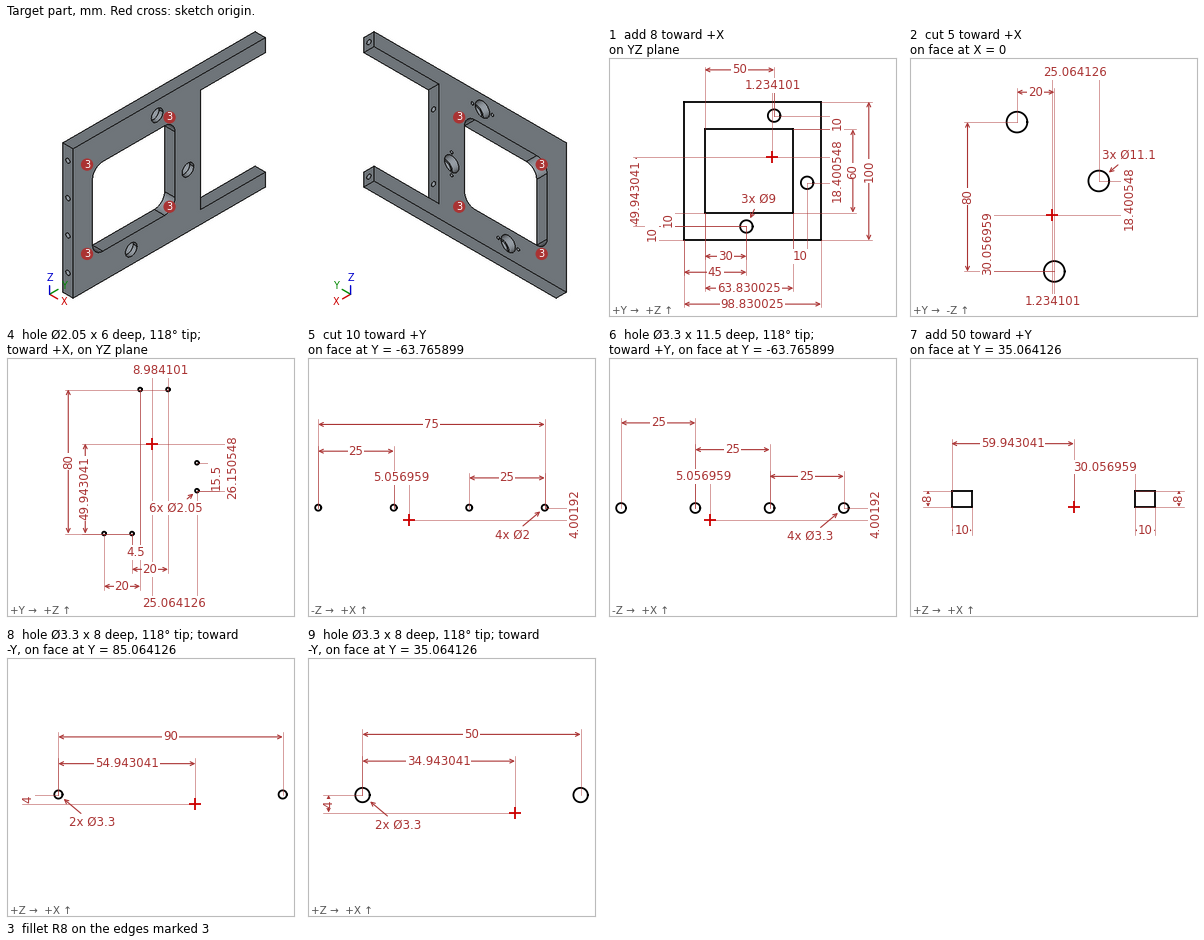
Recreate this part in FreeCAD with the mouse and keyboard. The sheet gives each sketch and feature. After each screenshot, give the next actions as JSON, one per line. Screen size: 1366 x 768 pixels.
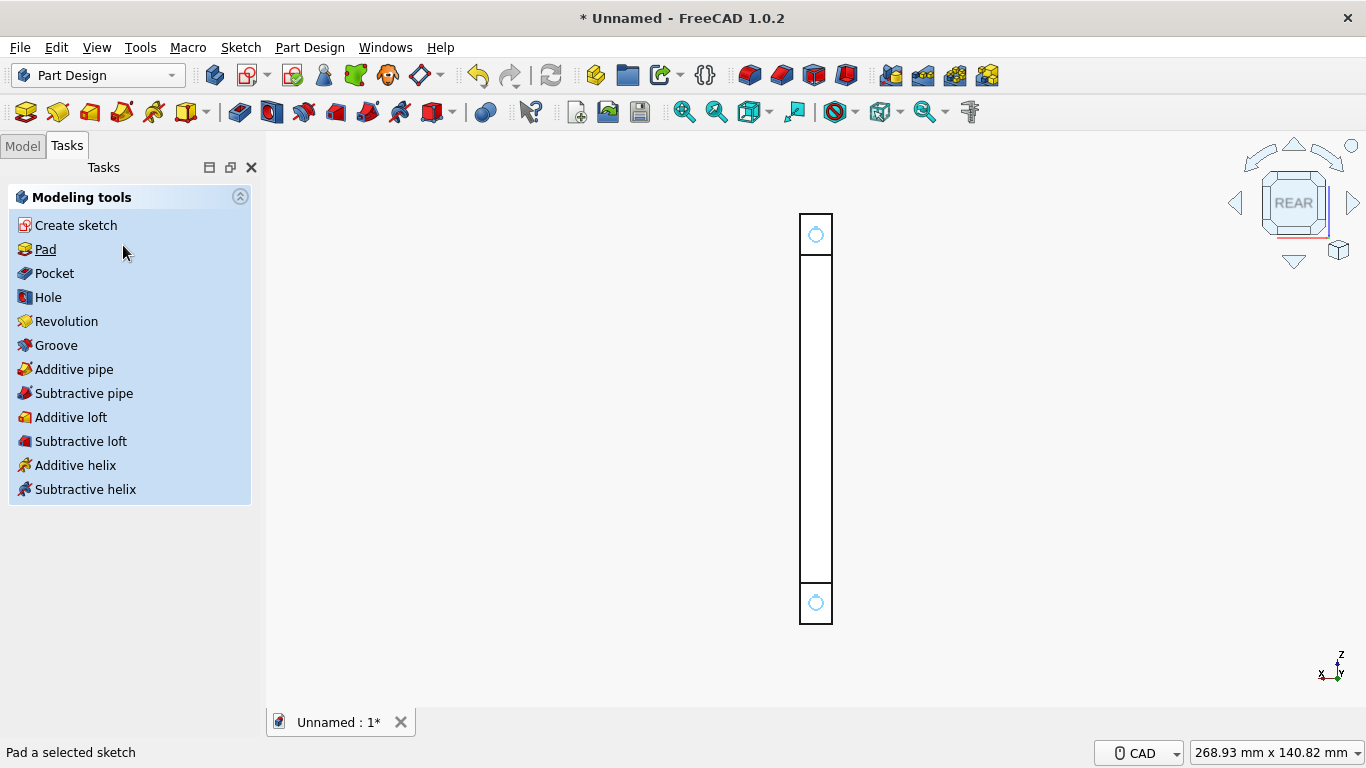
{"action": "left_click", "coordinate": [272, 112]}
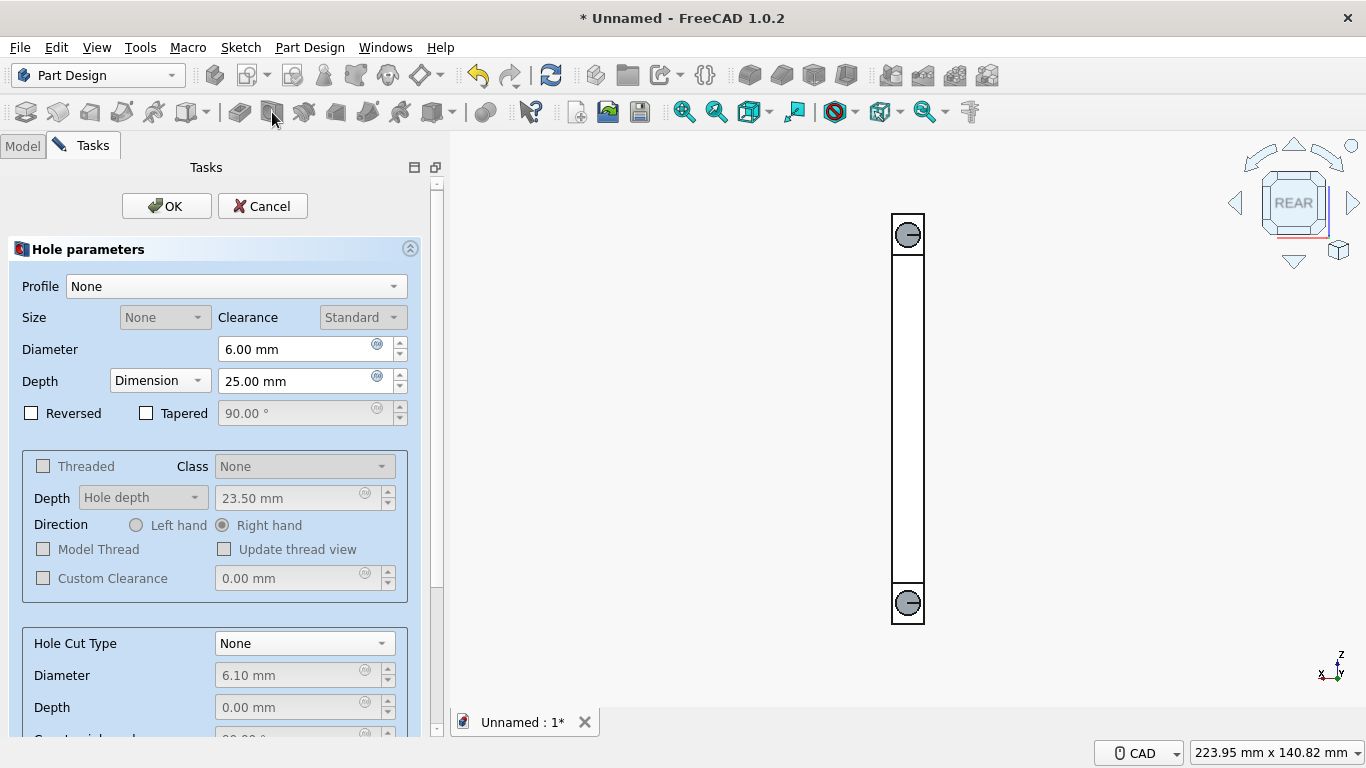
{"action": "triple_click", "coordinate": [305, 349]}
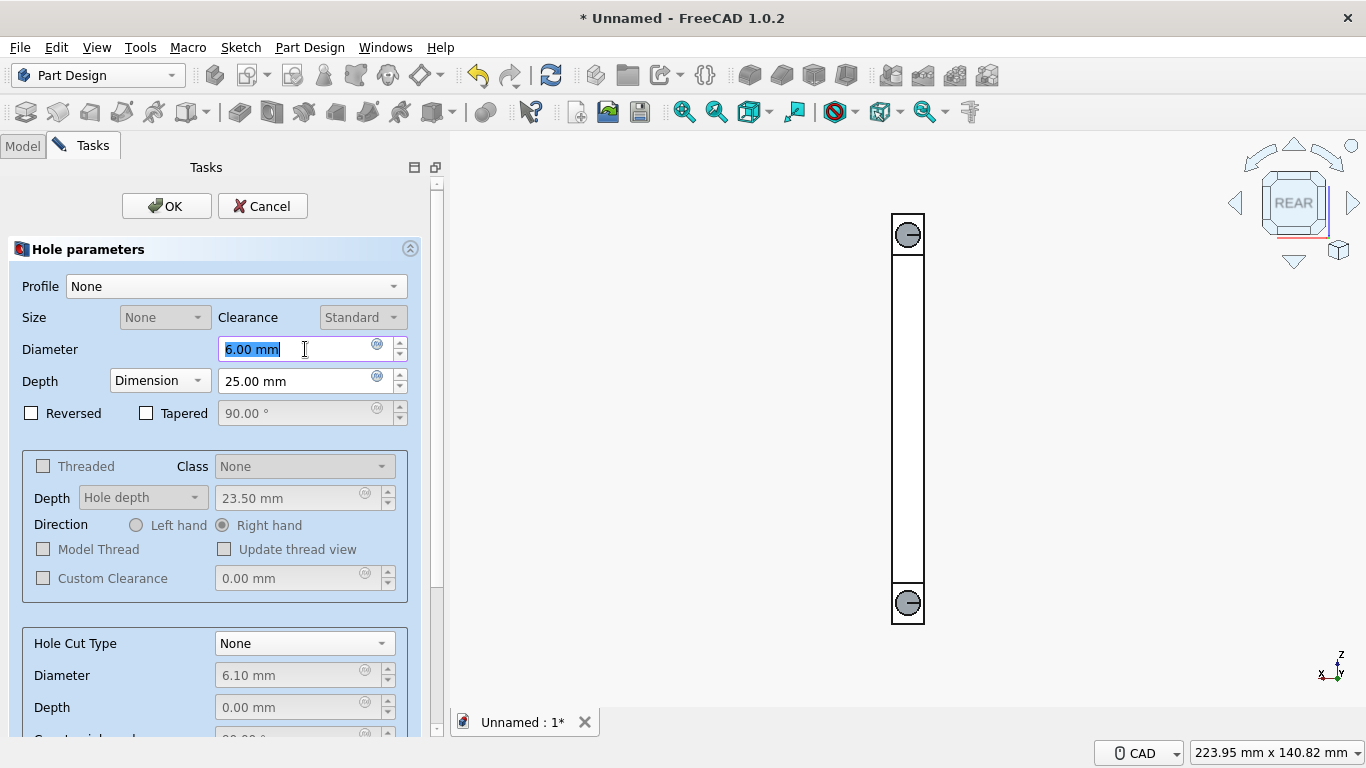
{"action": "type", "text": "3.3"}
{"action": "key", "text": "Tab"}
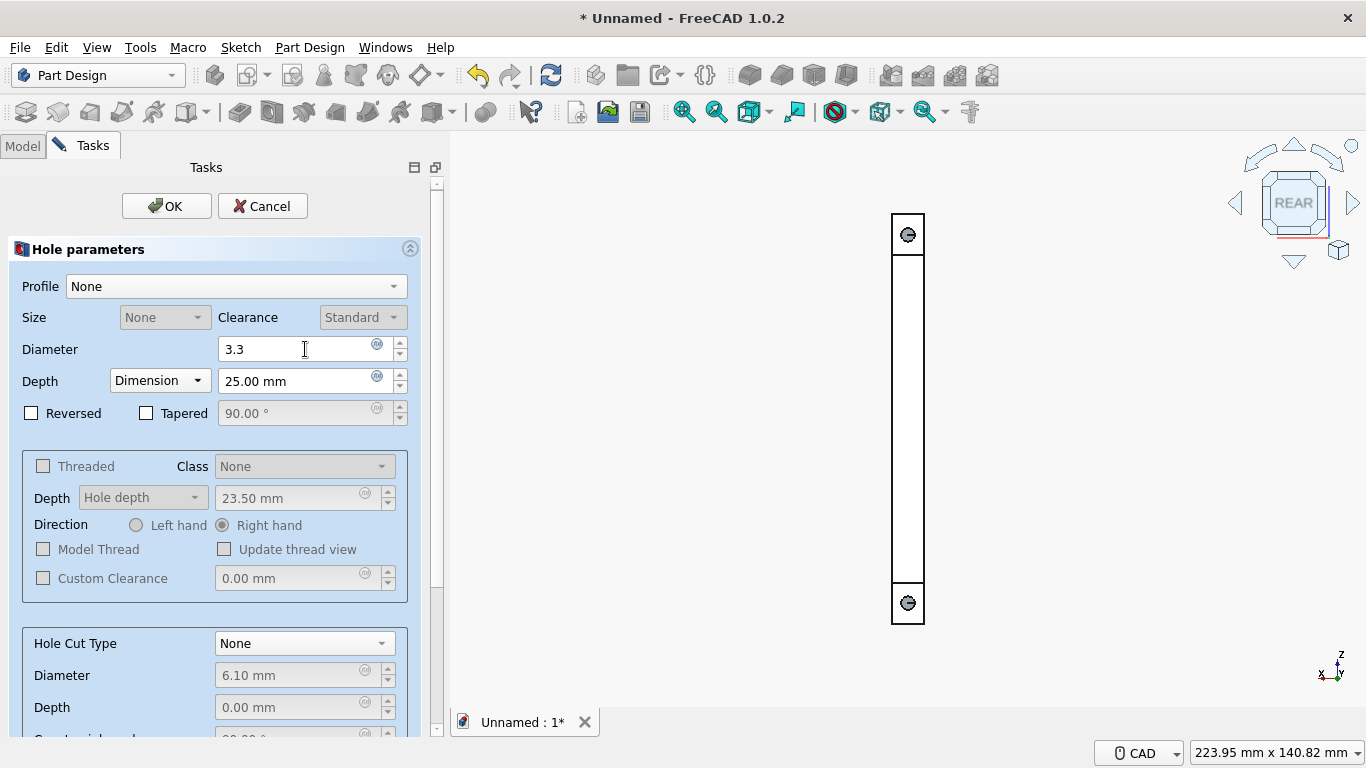
{"action": "triple_click", "coordinate": [305, 381]}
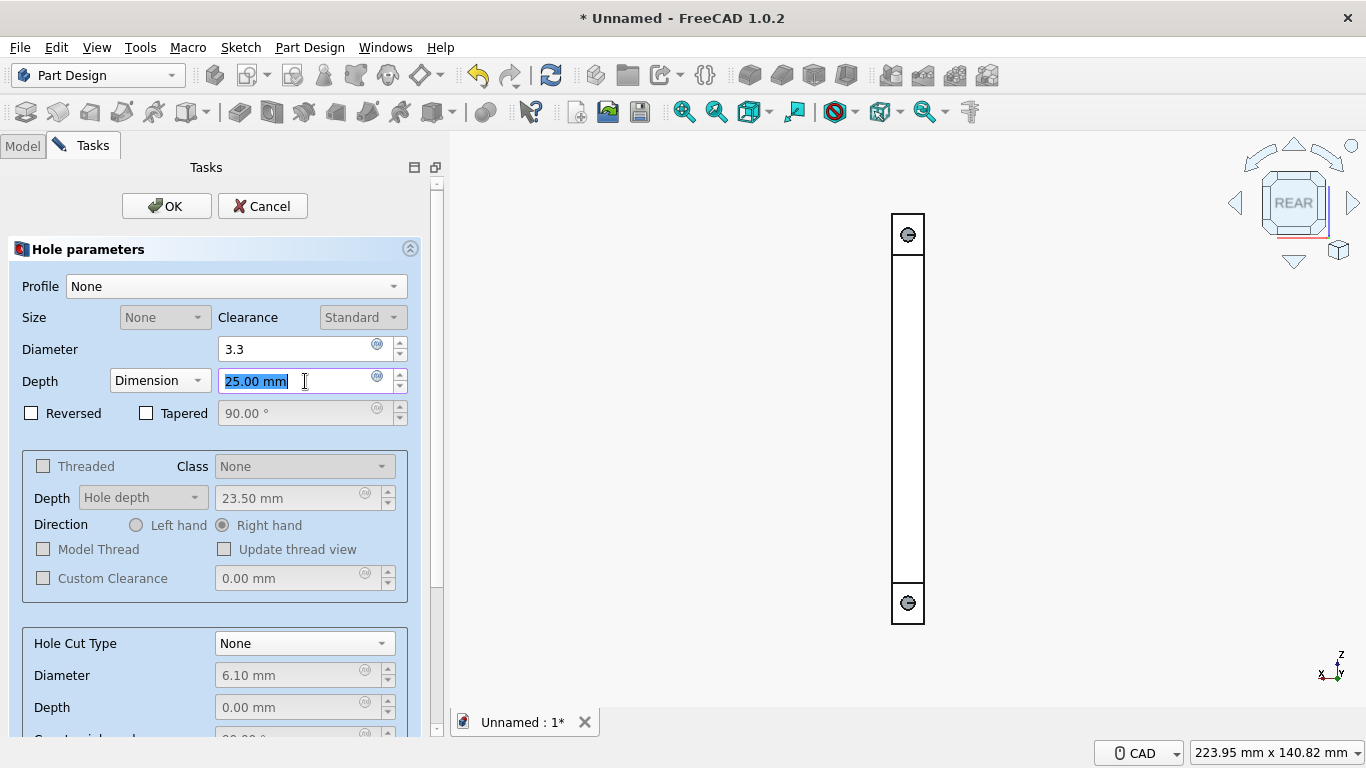
{"action": "type", "text": "8"}
{"action": "key", "text": "Tab"}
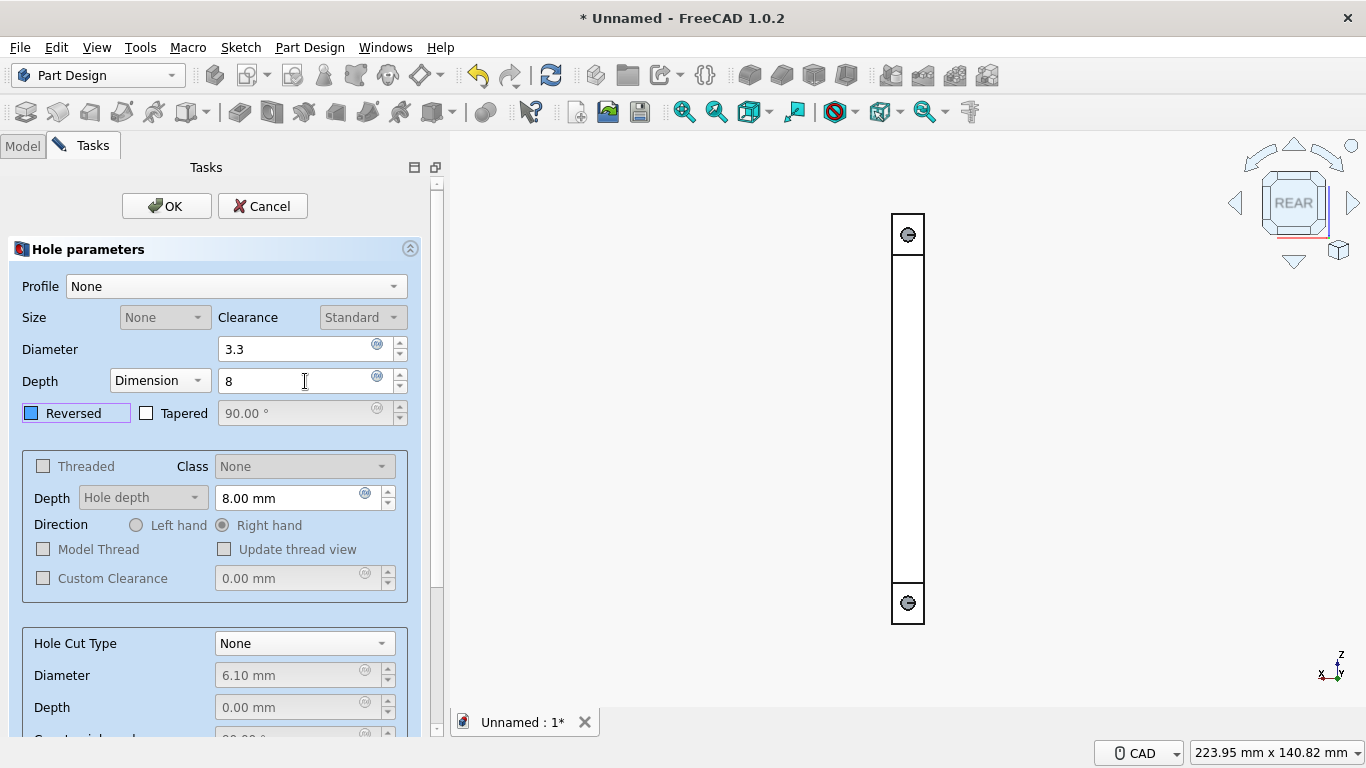
{"action": "left_click", "coordinate": [167, 206]}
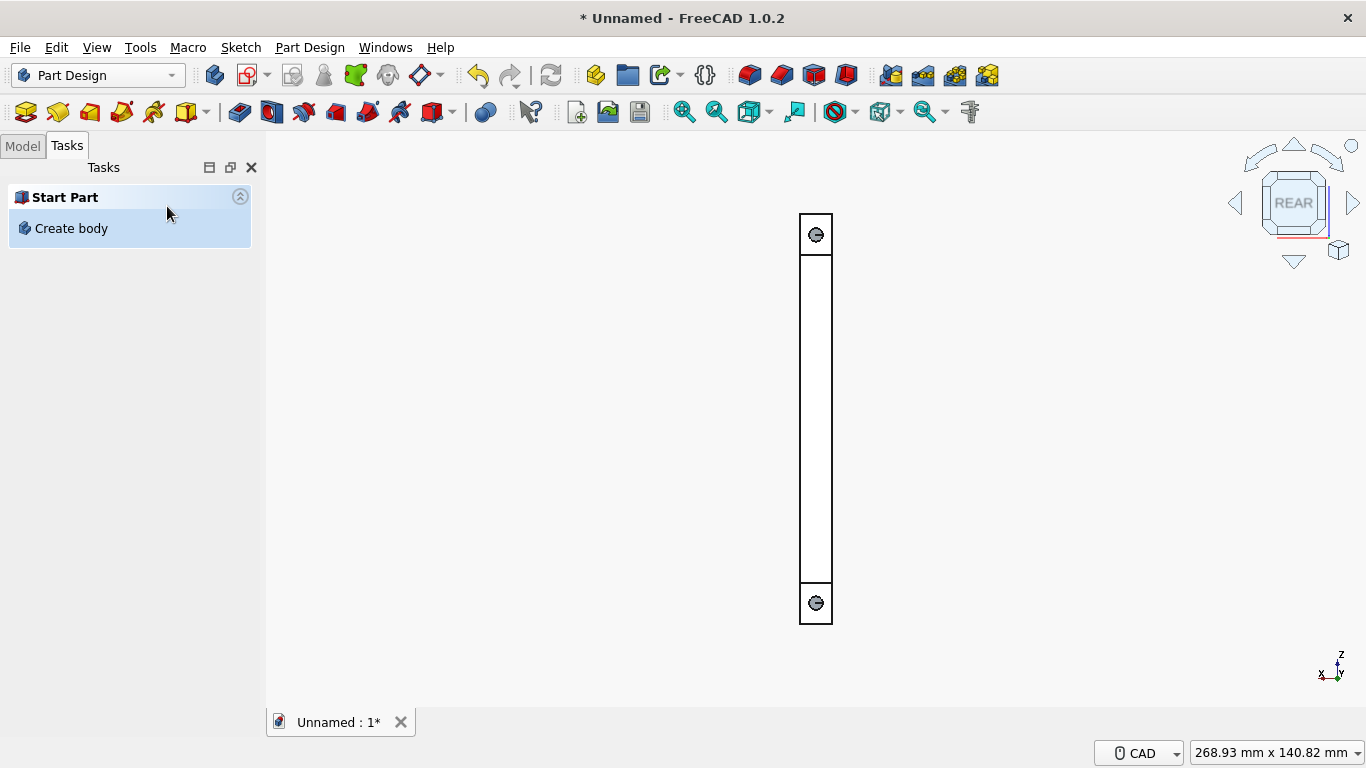
{"action": "left_click", "coordinate": [816, 325]}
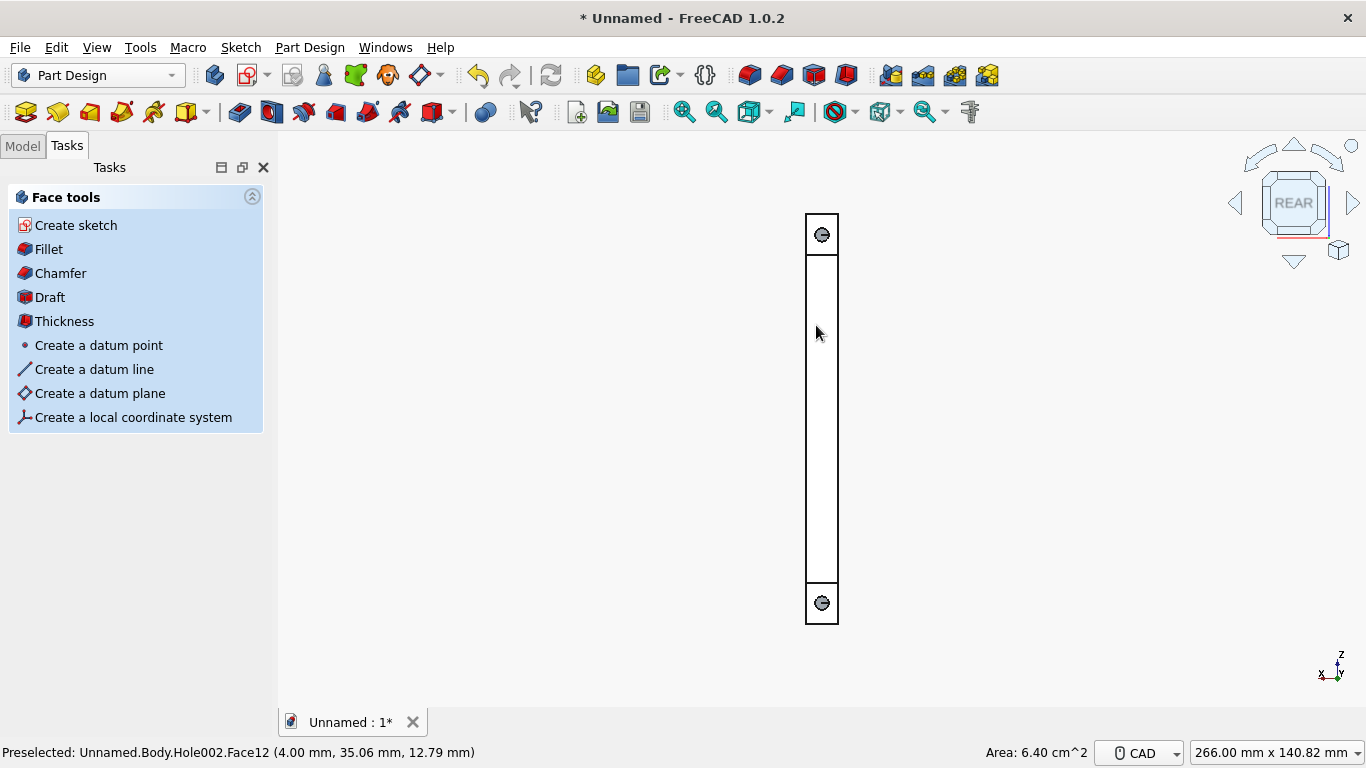
{"action": "left_click", "coordinate": [248, 76]}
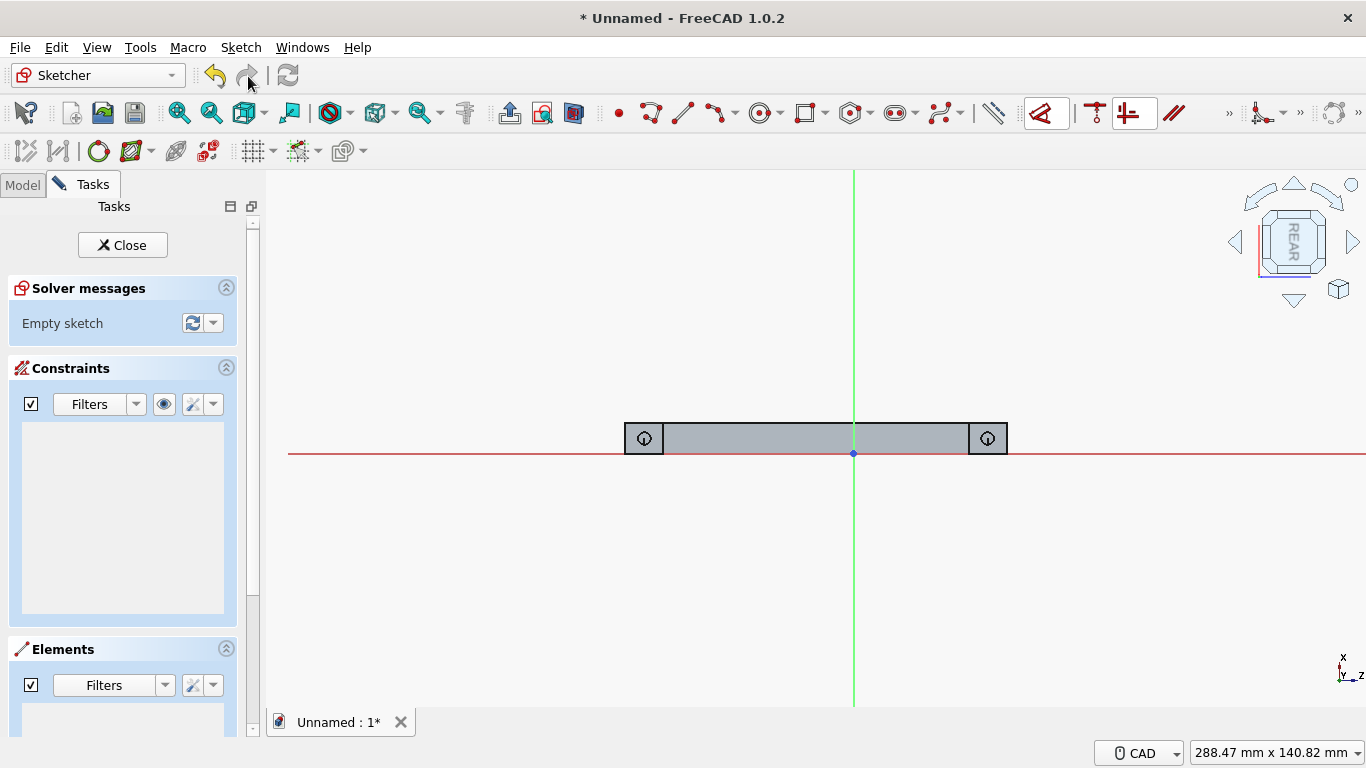
{"action": "scroll", "coordinate": [846, 445], "scroll_direction": "up", "scroll_amount": 6}